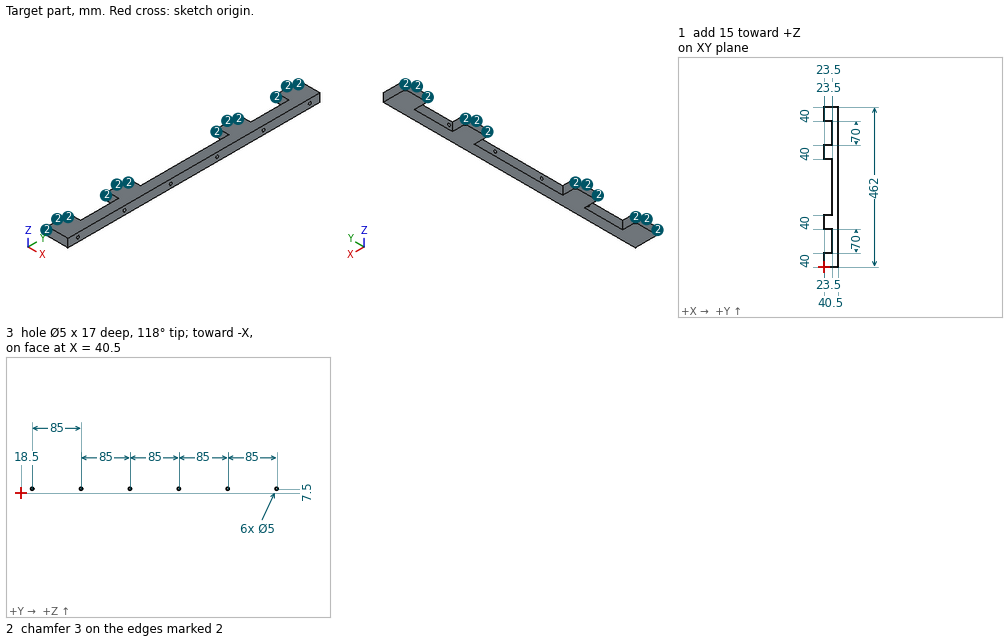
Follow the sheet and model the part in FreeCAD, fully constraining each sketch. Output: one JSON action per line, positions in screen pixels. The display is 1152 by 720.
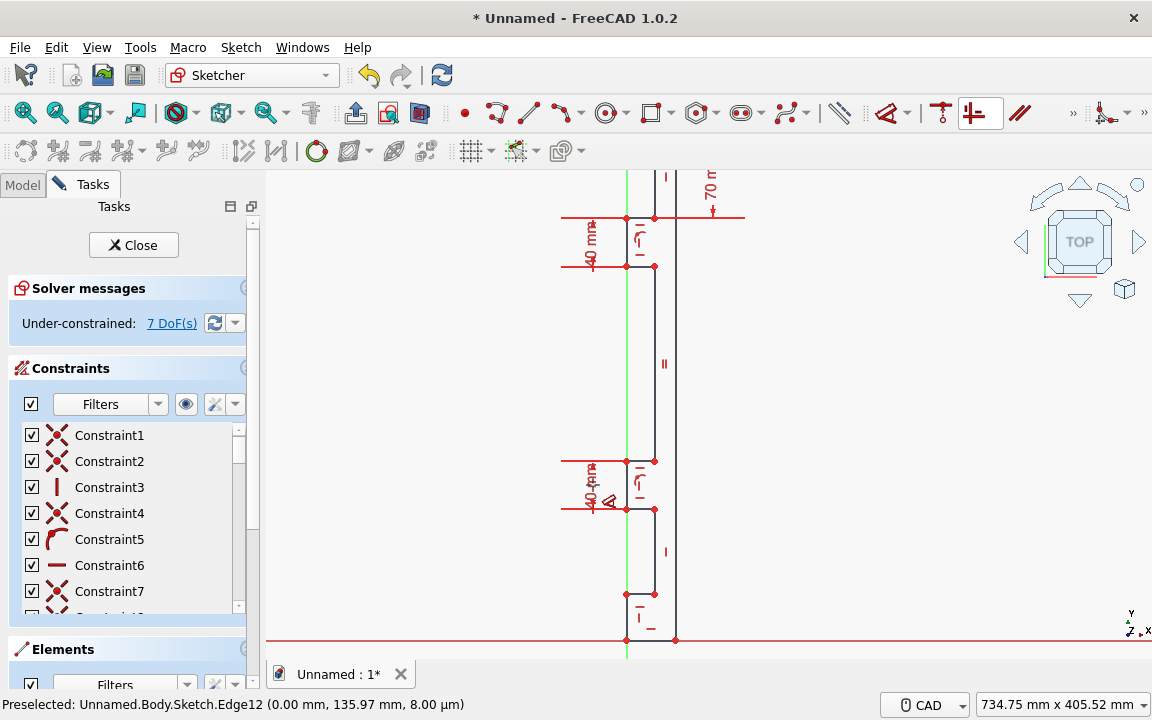
{"action": "left_click", "coordinate": [655, 535]}
{"action": "left_click", "coordinate": [713, 552]}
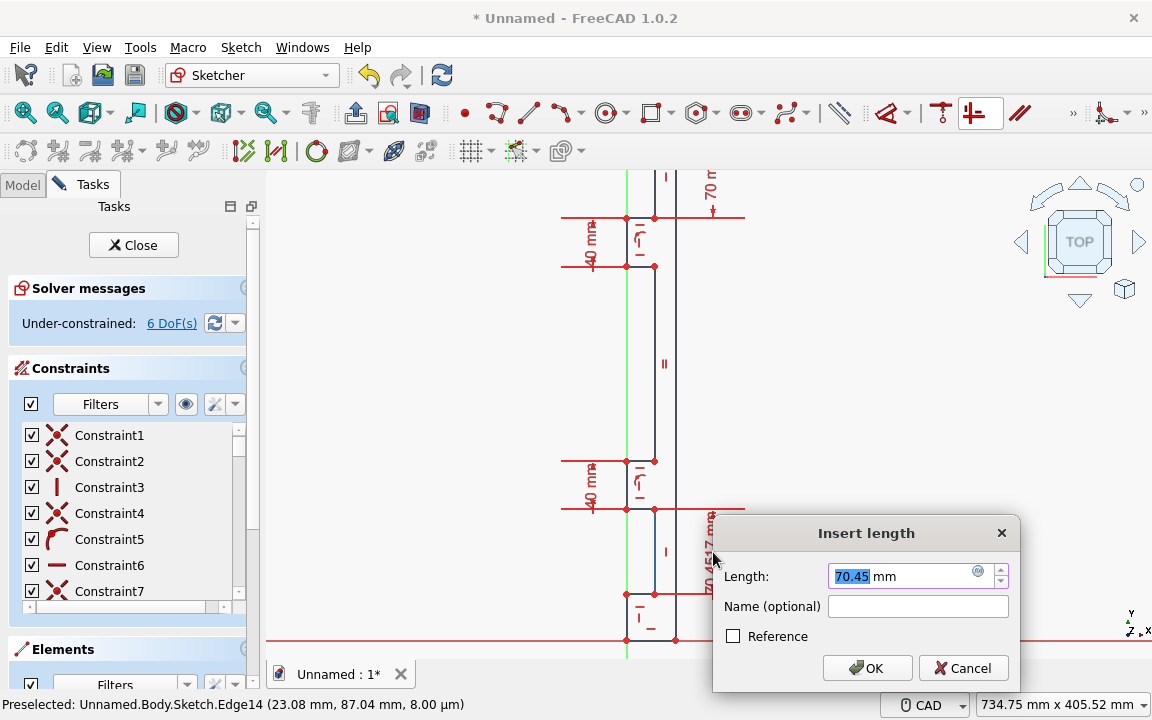
{"action": "type", "text": "70"}
{"action": "key", "text": "Return"}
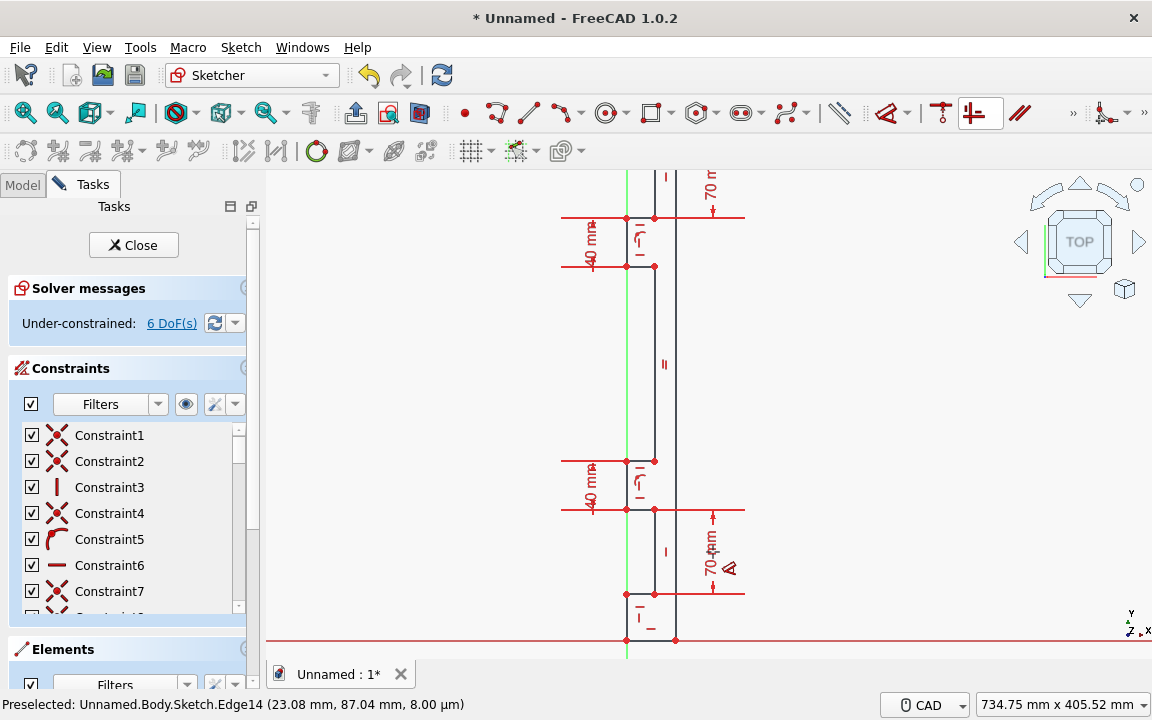
{"action": "left_click", "coordinate": [627, 608]}
{"action": "left_click", "coordinate": [593, 613]}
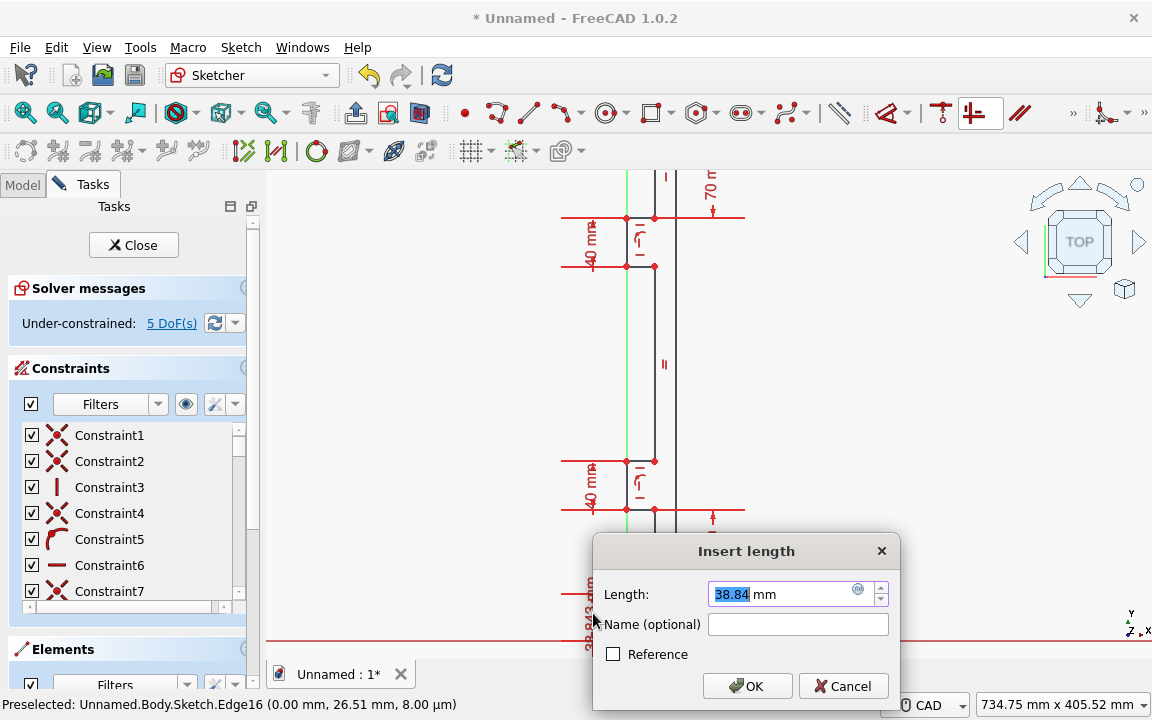
{"action": "type", "text": "40"}
{"action": "key", "text": "Return"}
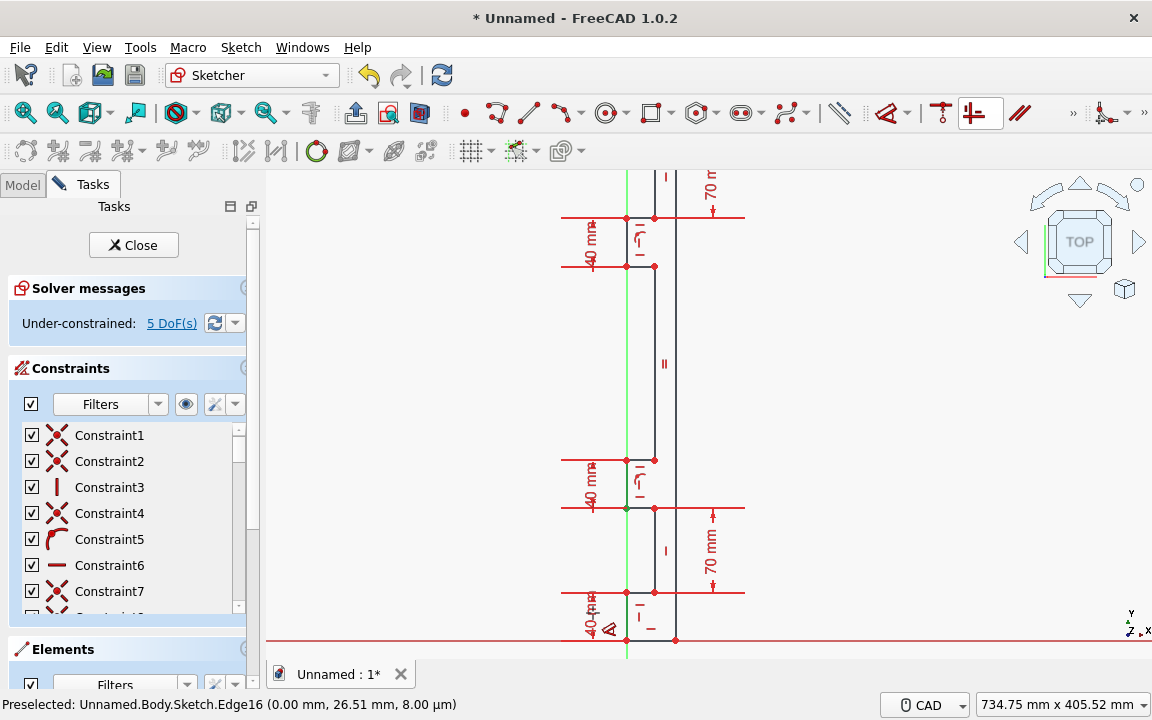
{"action": "left_click", "coordinate": [676, 474]}
{"action": "left_click", "coordinate": [710, 414]}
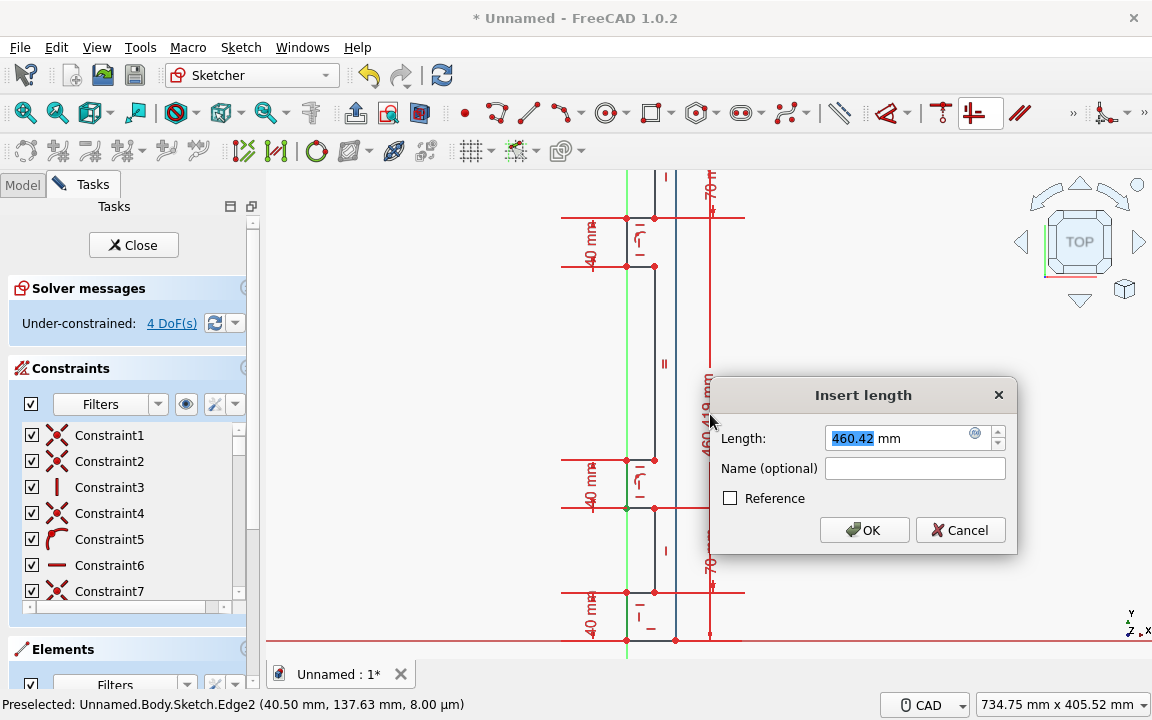
{"action": "type", "text": "462"}
{"action": "key", "text": "Return"}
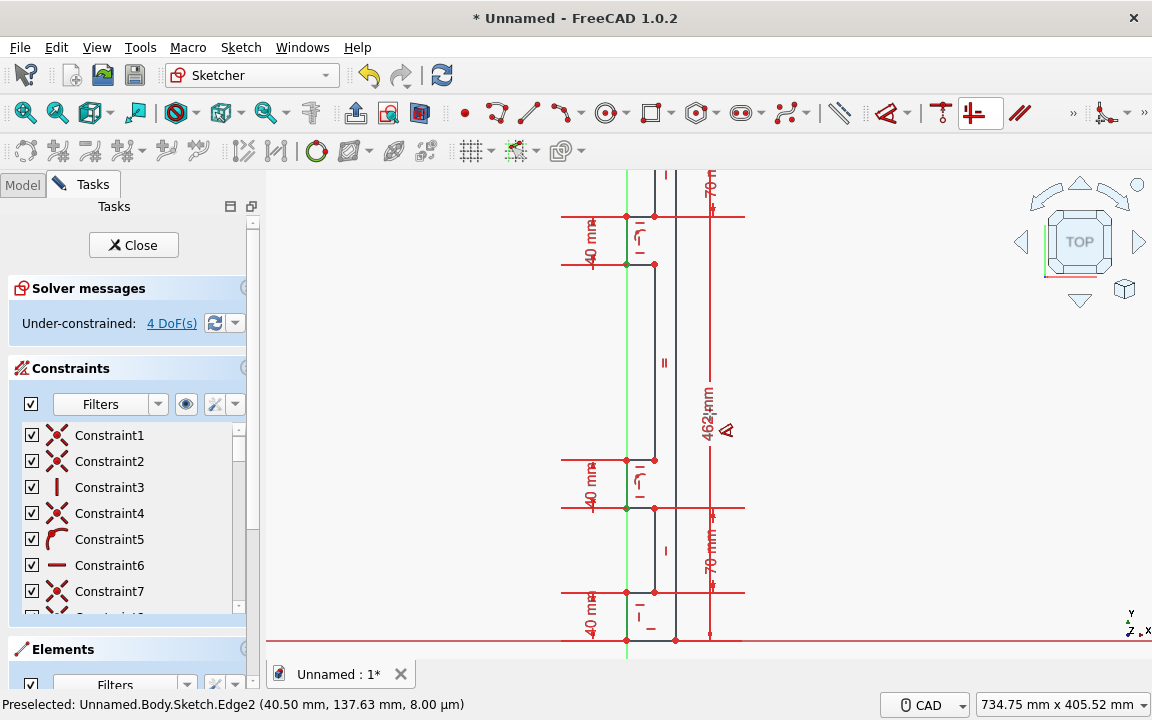
{"action": "scroll", "coordinate": [627, 478], "scroll_direction": "down", "scroll_amount": 3}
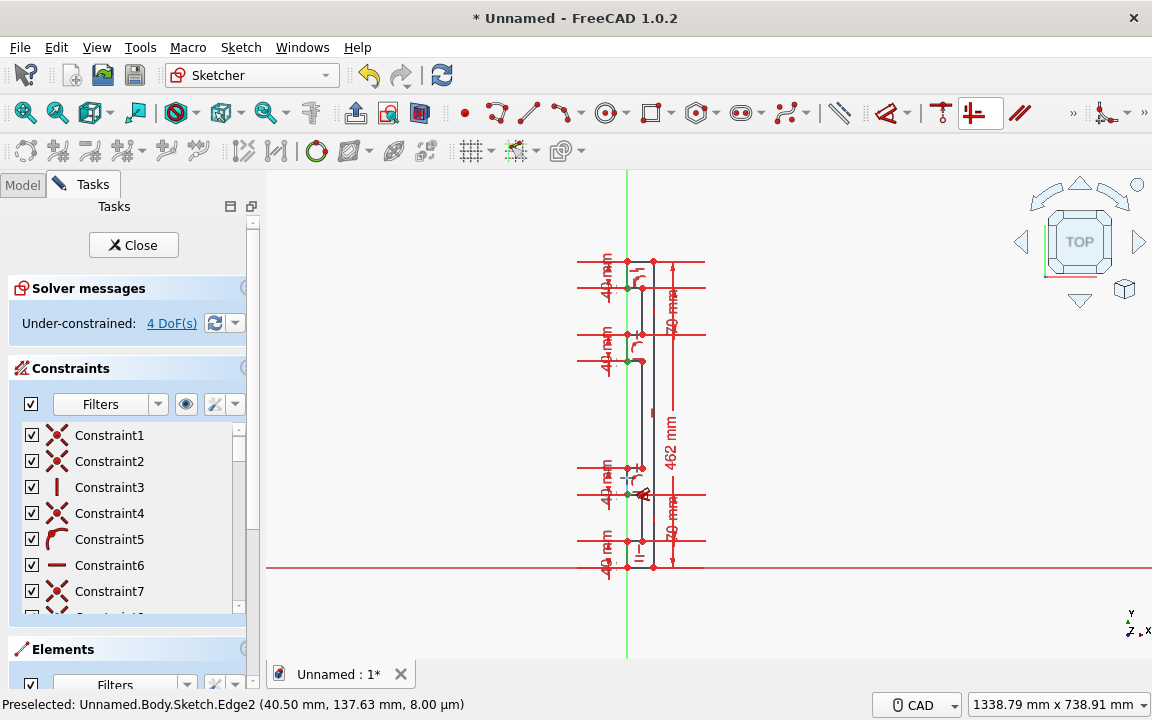
{"action": "scroll", "coordinate": [635, 568], "scroll_direction": "up", "scroll_amount": 3}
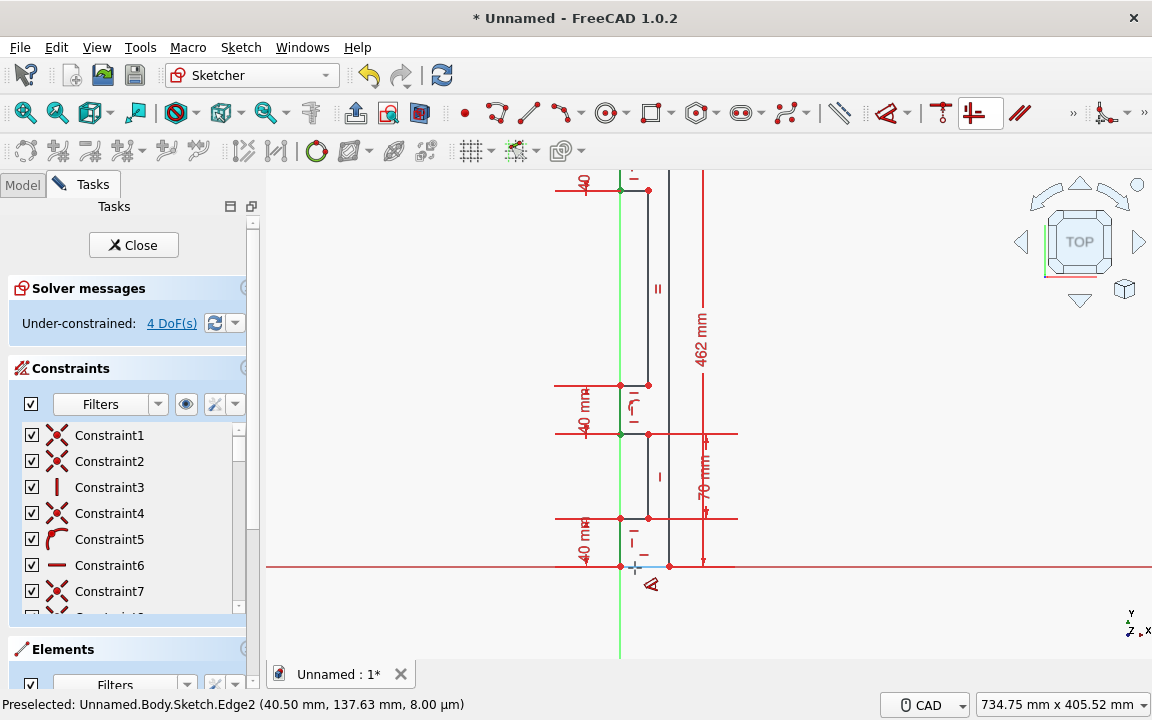
{"action": "left_click", "coordinate": [635, 567]}
{"action": "left_click", "coordinate": [645, 601]}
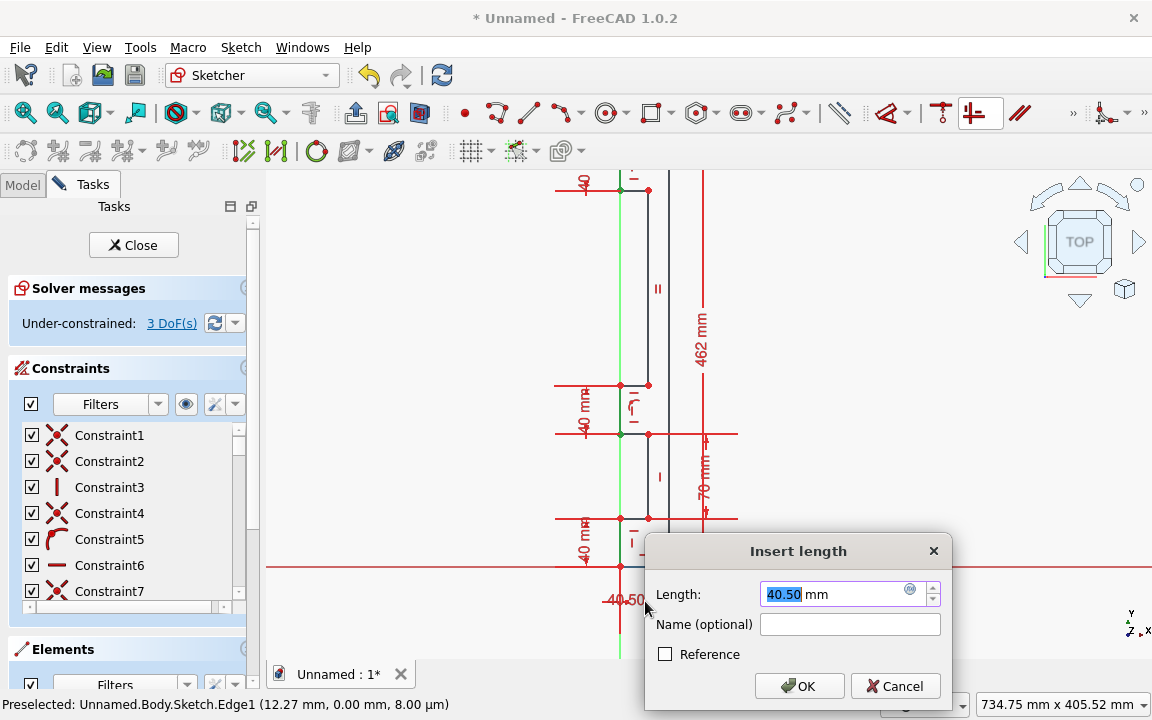
{"action": "type", "text": "40.5"}
{"action": "key", "text": "Return"}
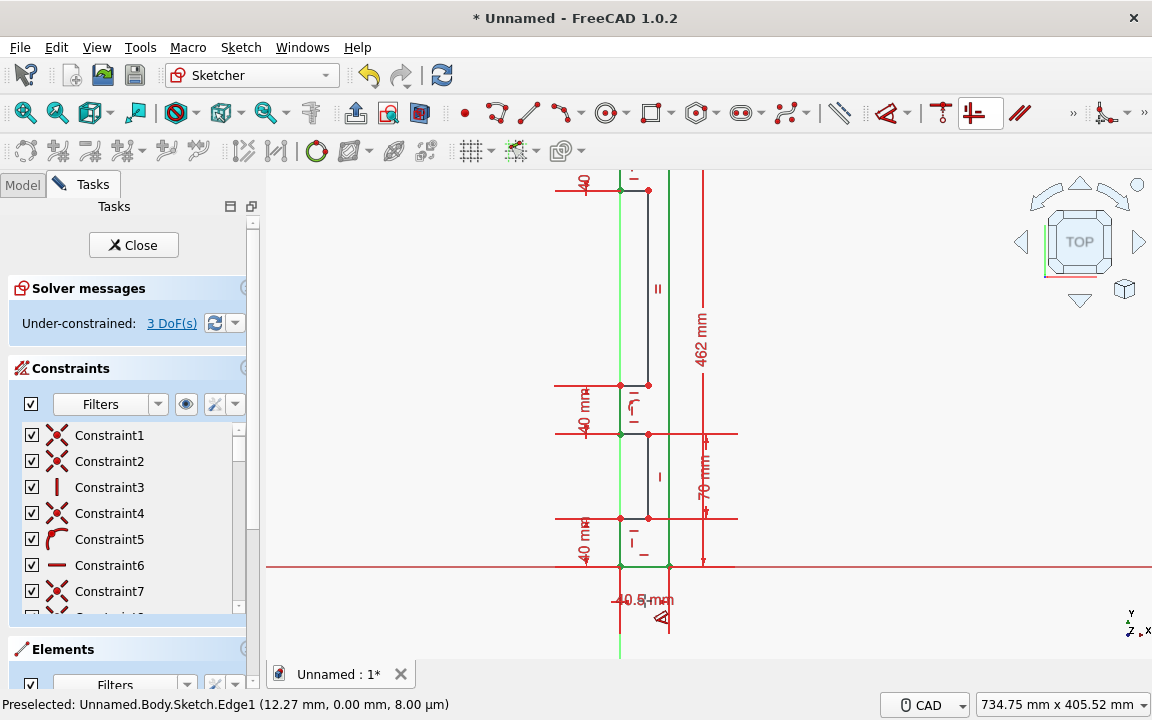
{"action": "scroll", "coordinate": [635, 568], "scroll_direction": "down", "scroll_amount": 3}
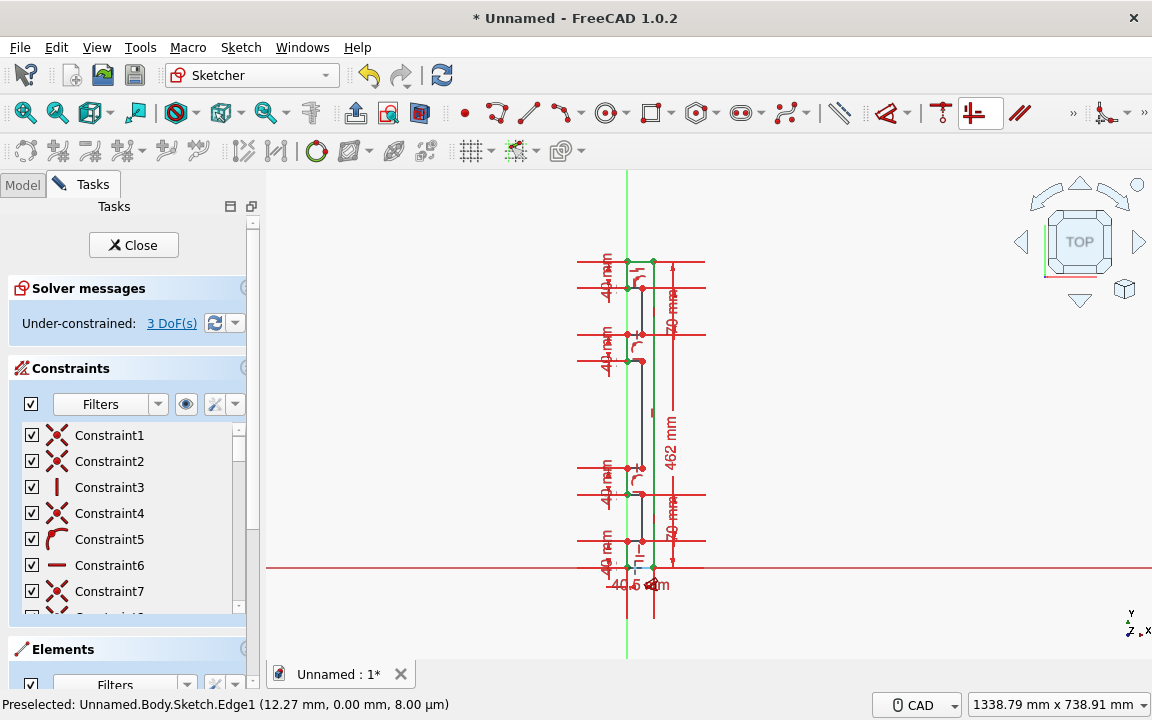
{"action": "scroll", "coordinate": [633, 288], "scroll_direction": "up", "scroll_amount": 5}